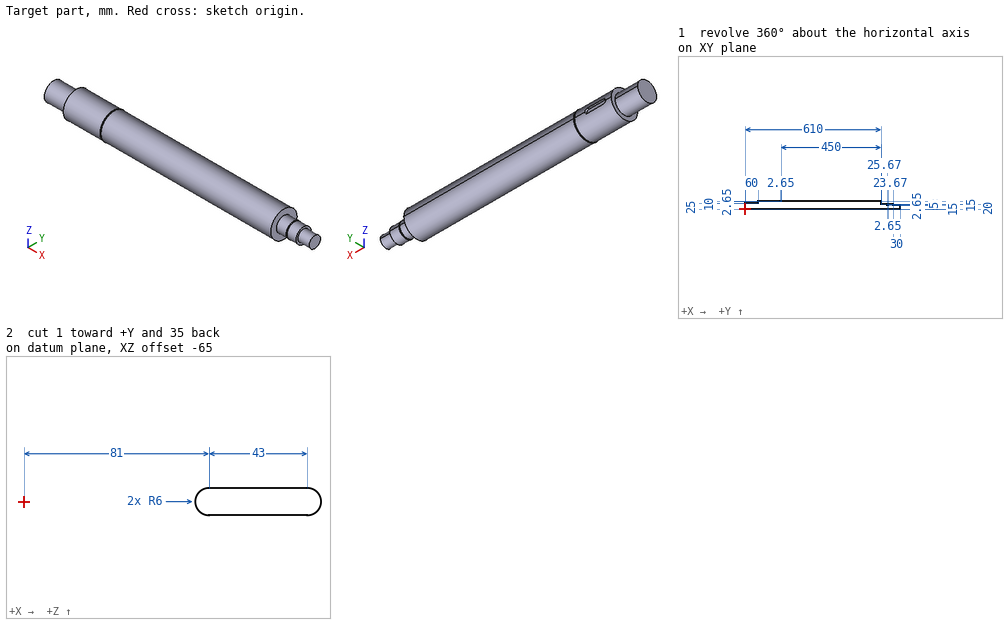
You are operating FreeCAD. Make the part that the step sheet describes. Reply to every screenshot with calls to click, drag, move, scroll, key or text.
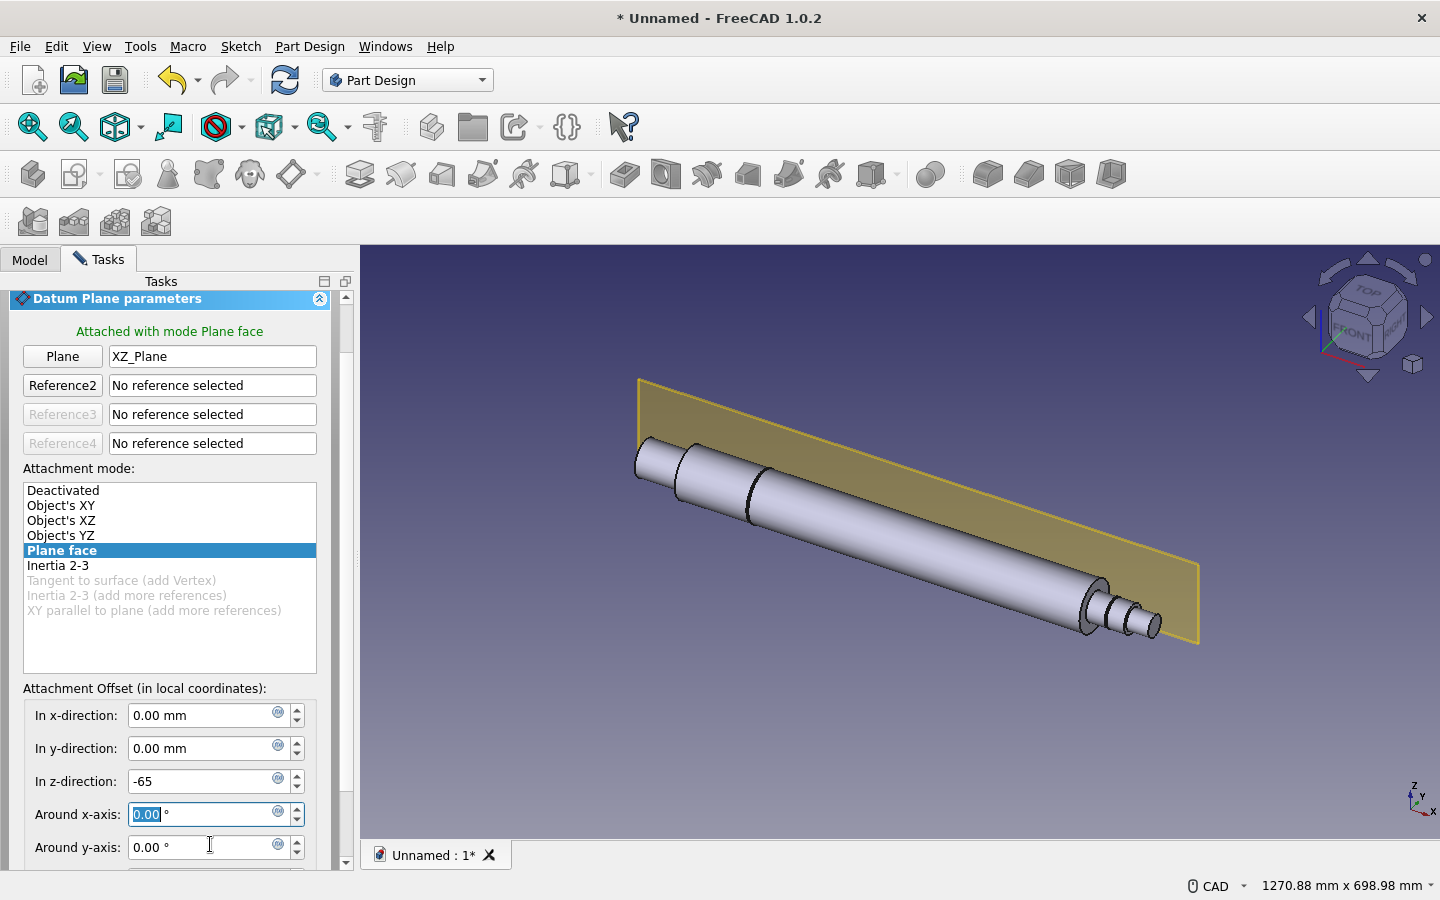
scroll(346, 580, up, 2)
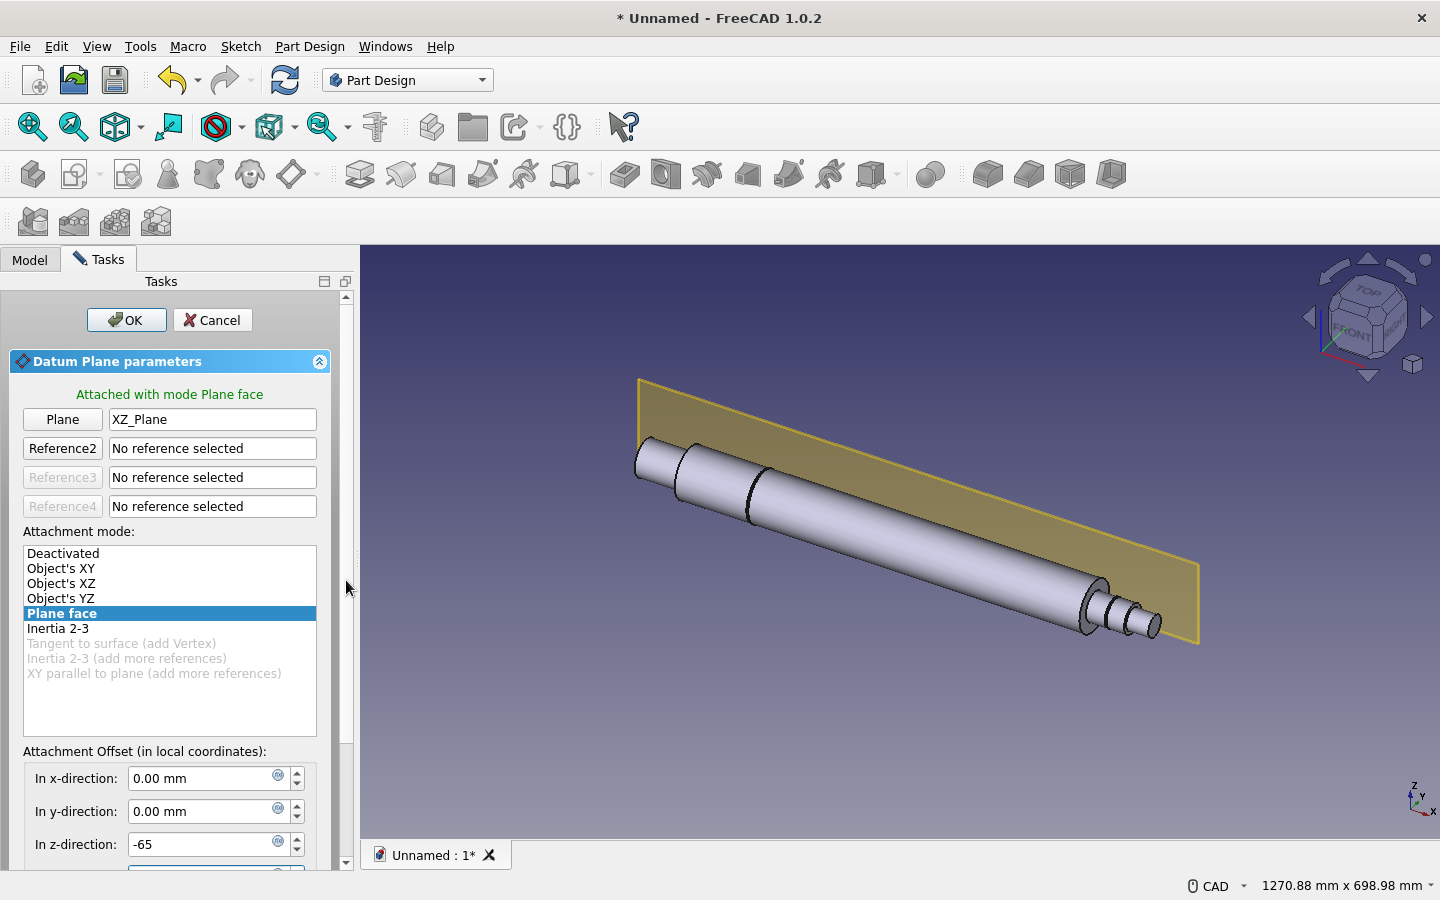
click(127, 320)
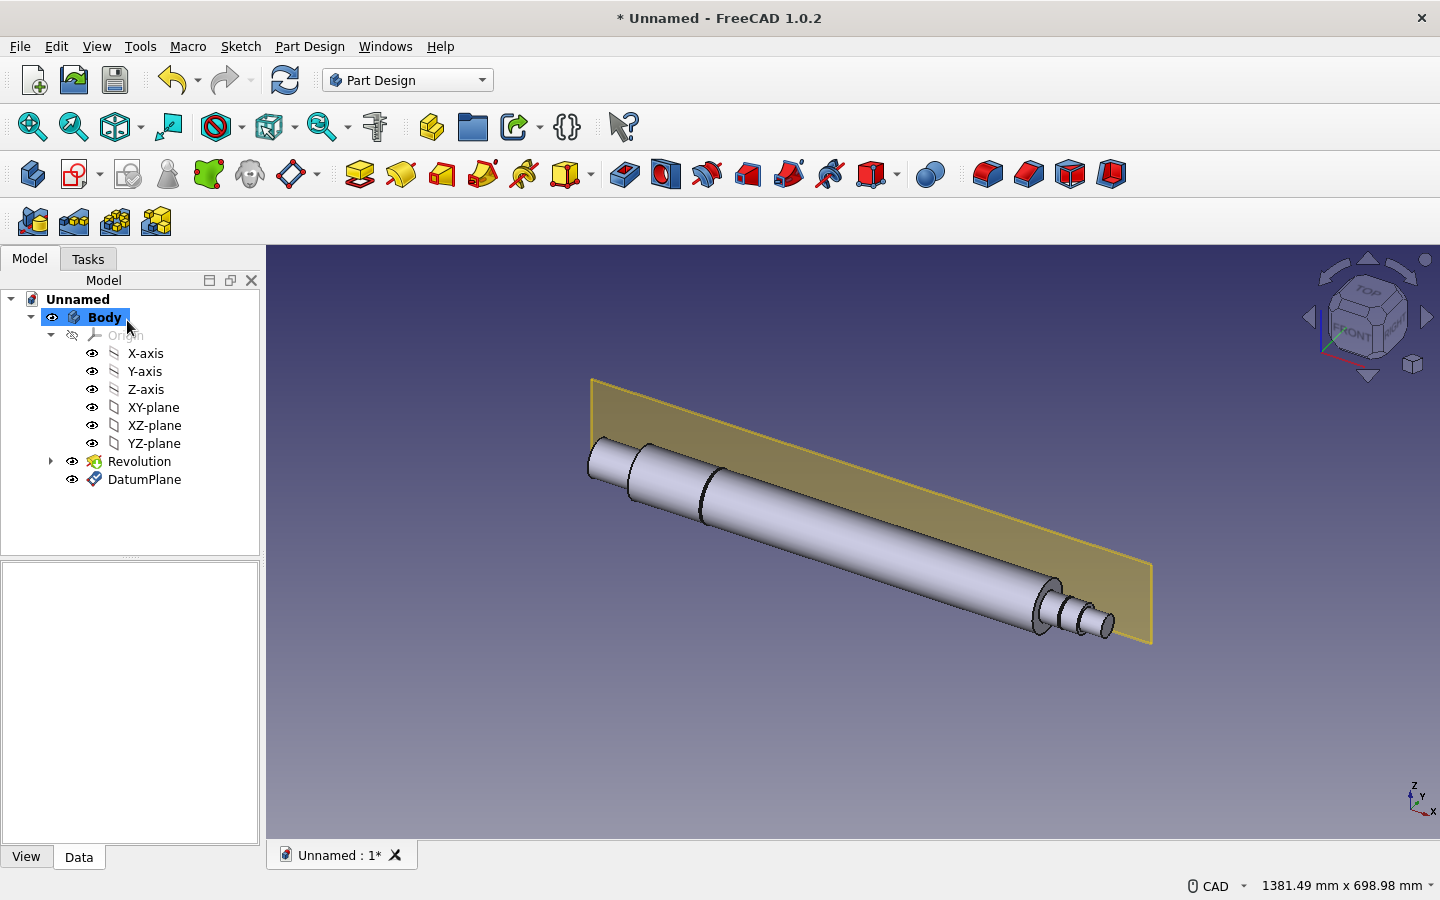
click(117, 479)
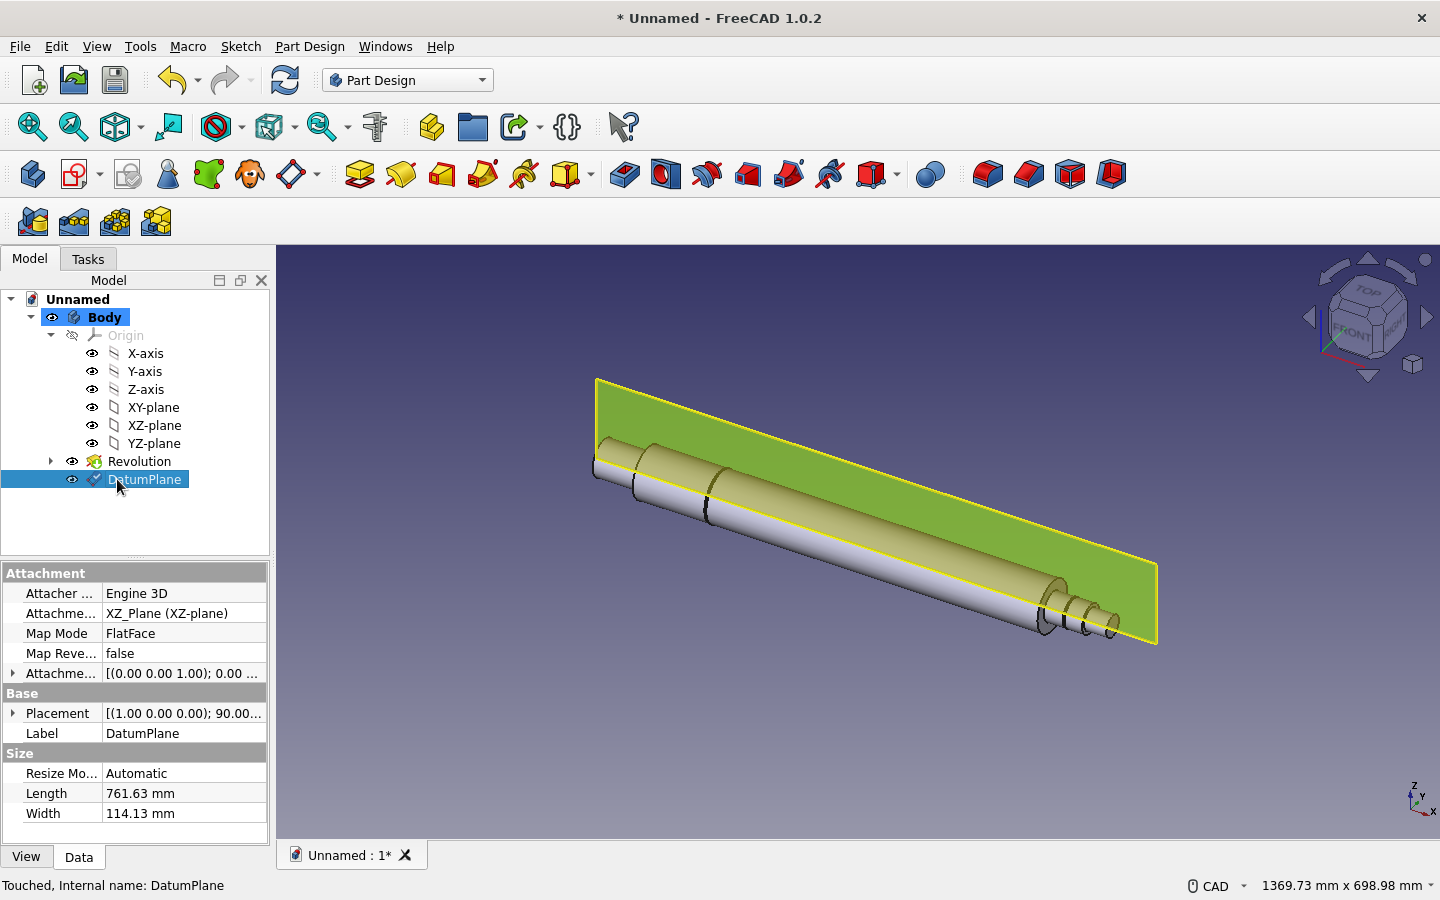
click(74, 174)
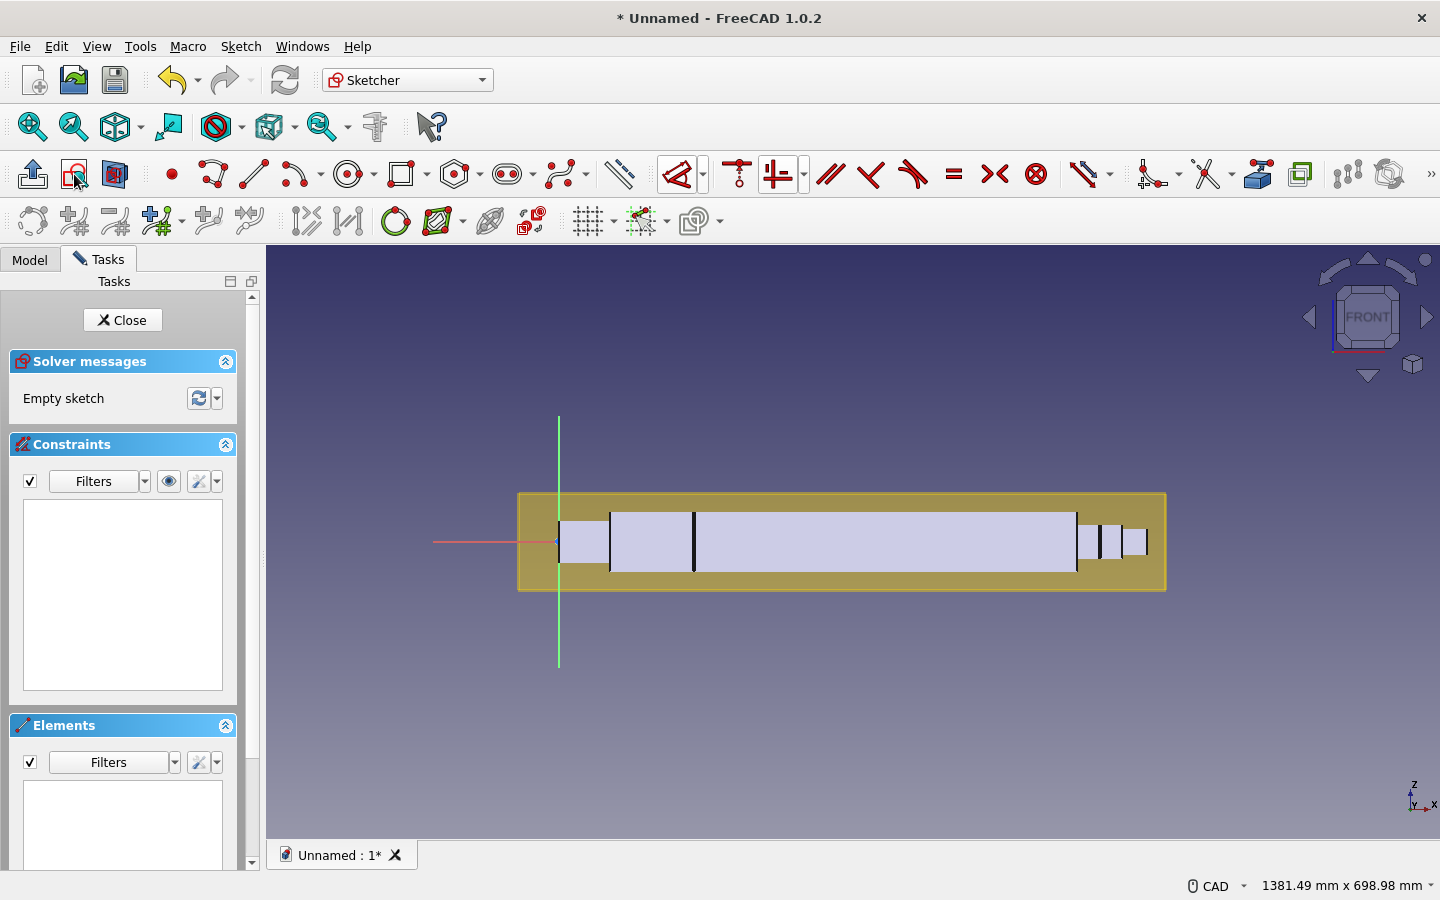
key(q)
key(s)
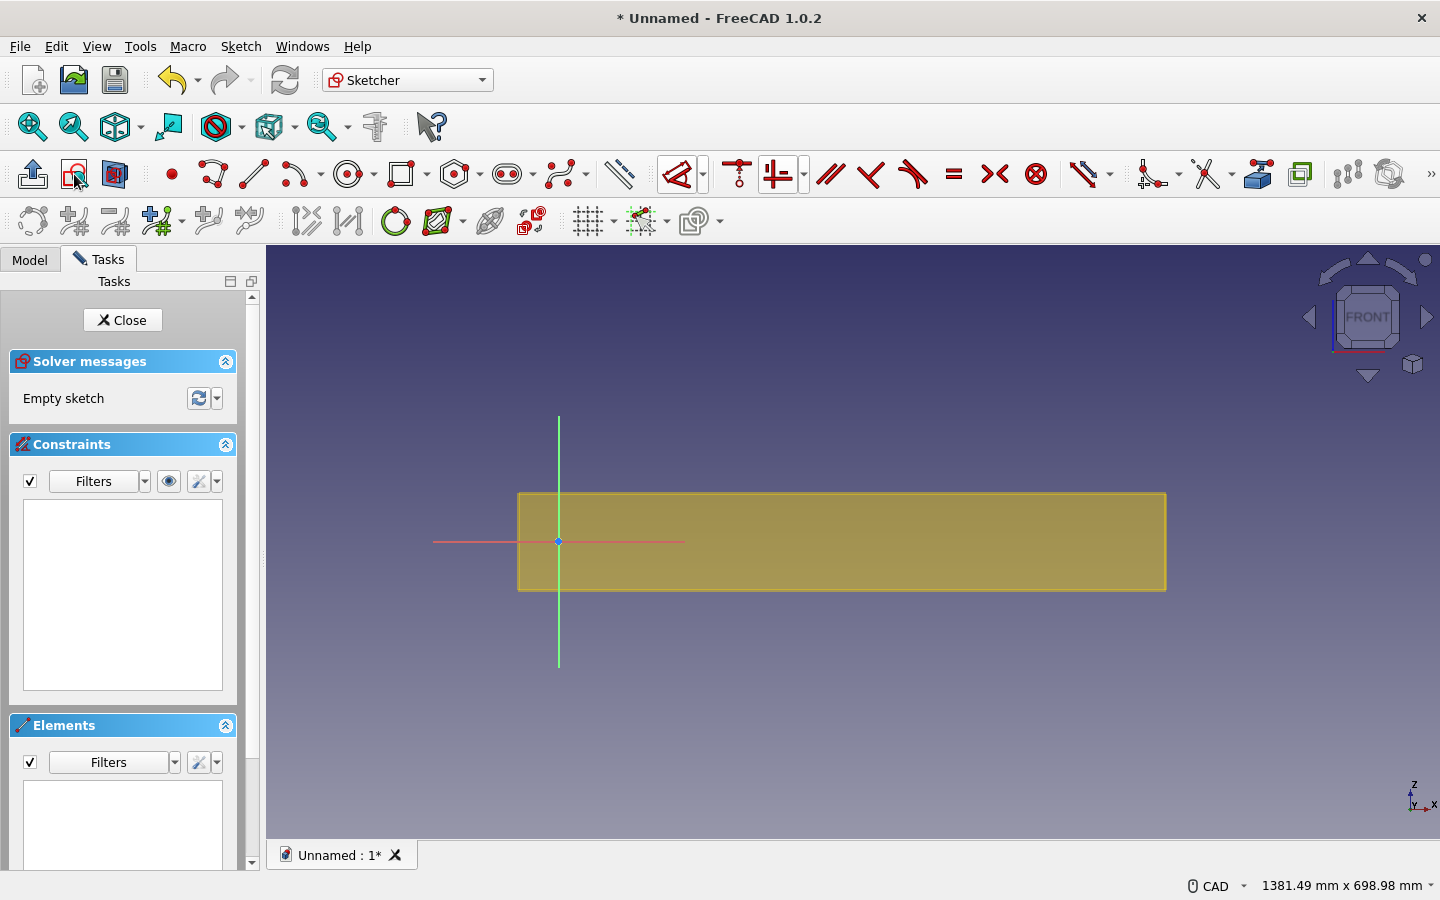
scroll(580, 542, up, 9)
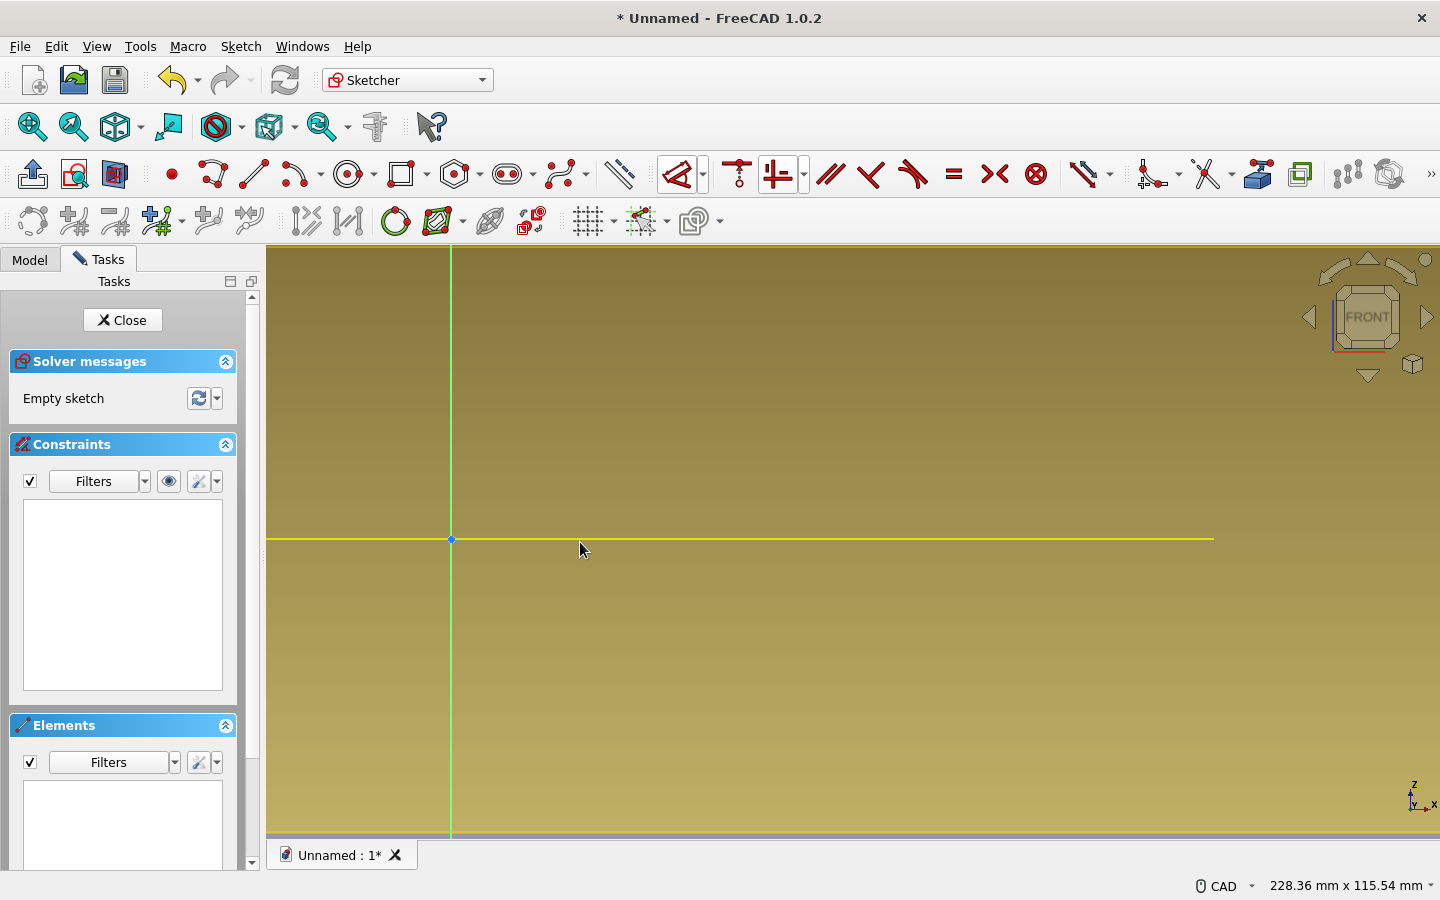
click(506, 174)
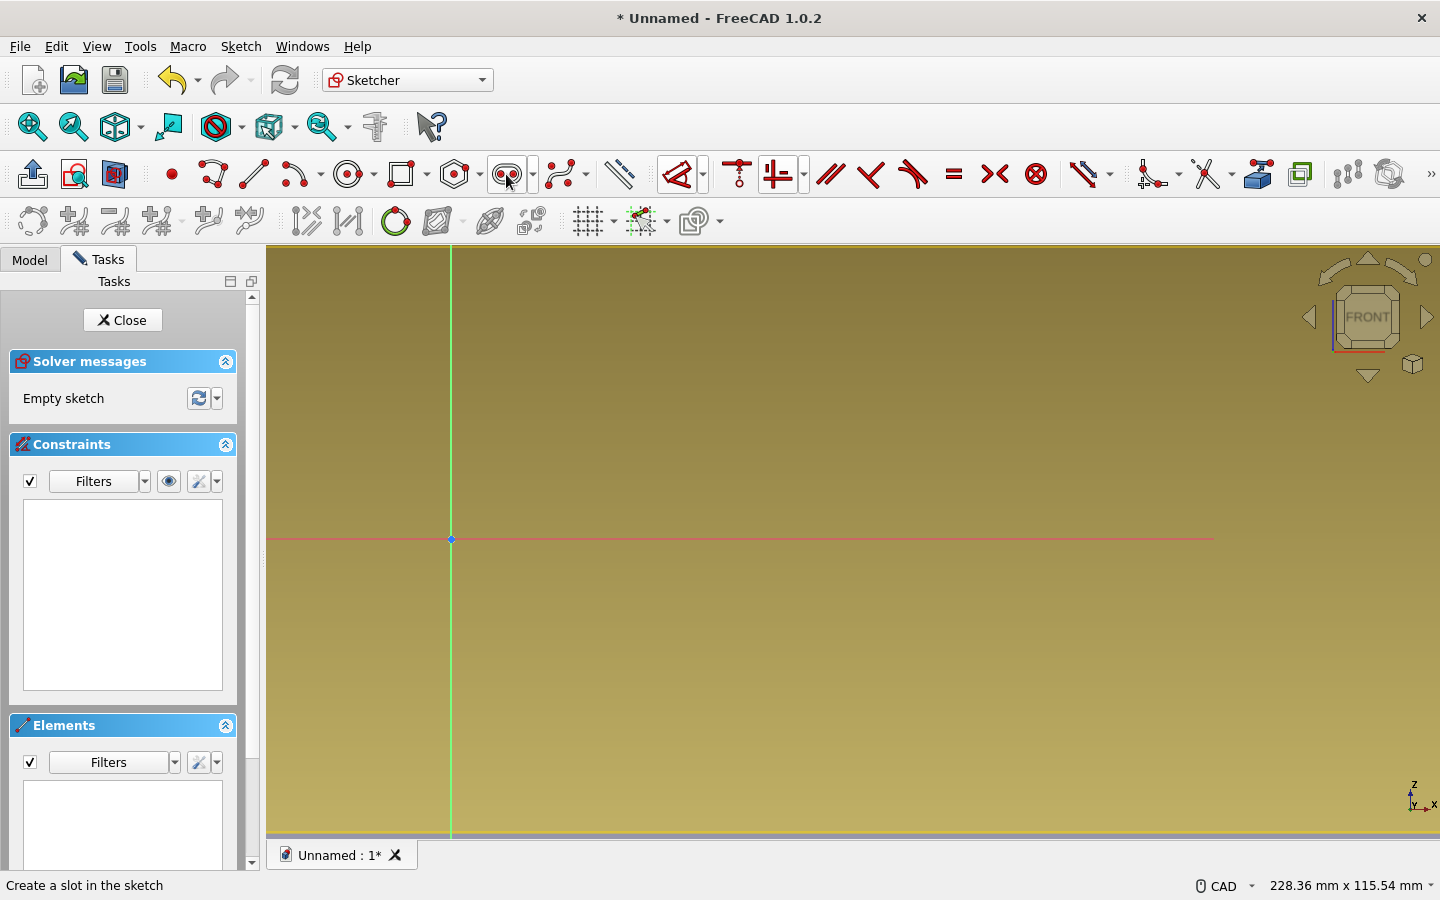
click(868, 539)